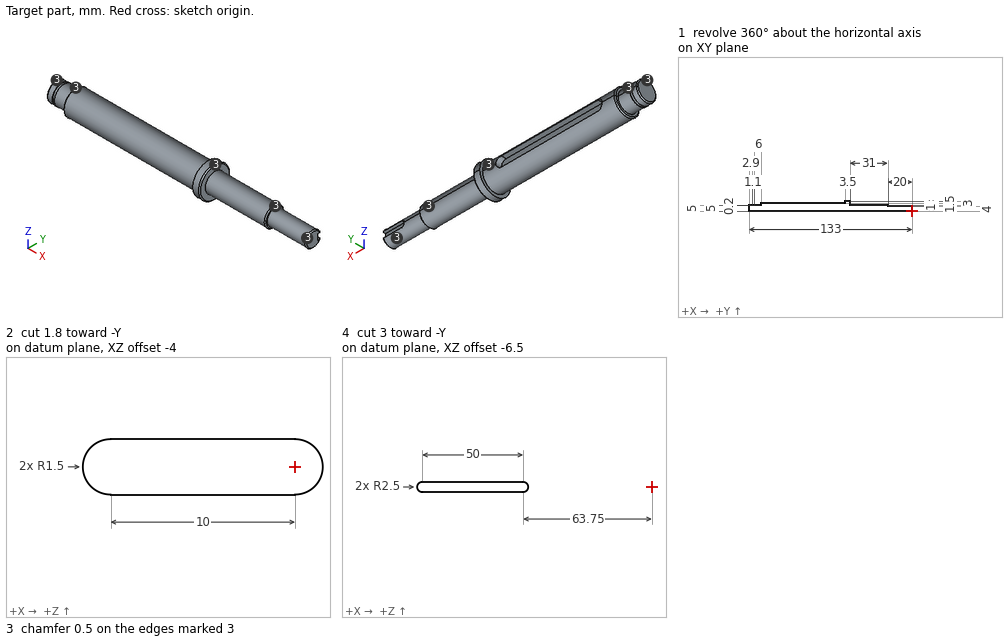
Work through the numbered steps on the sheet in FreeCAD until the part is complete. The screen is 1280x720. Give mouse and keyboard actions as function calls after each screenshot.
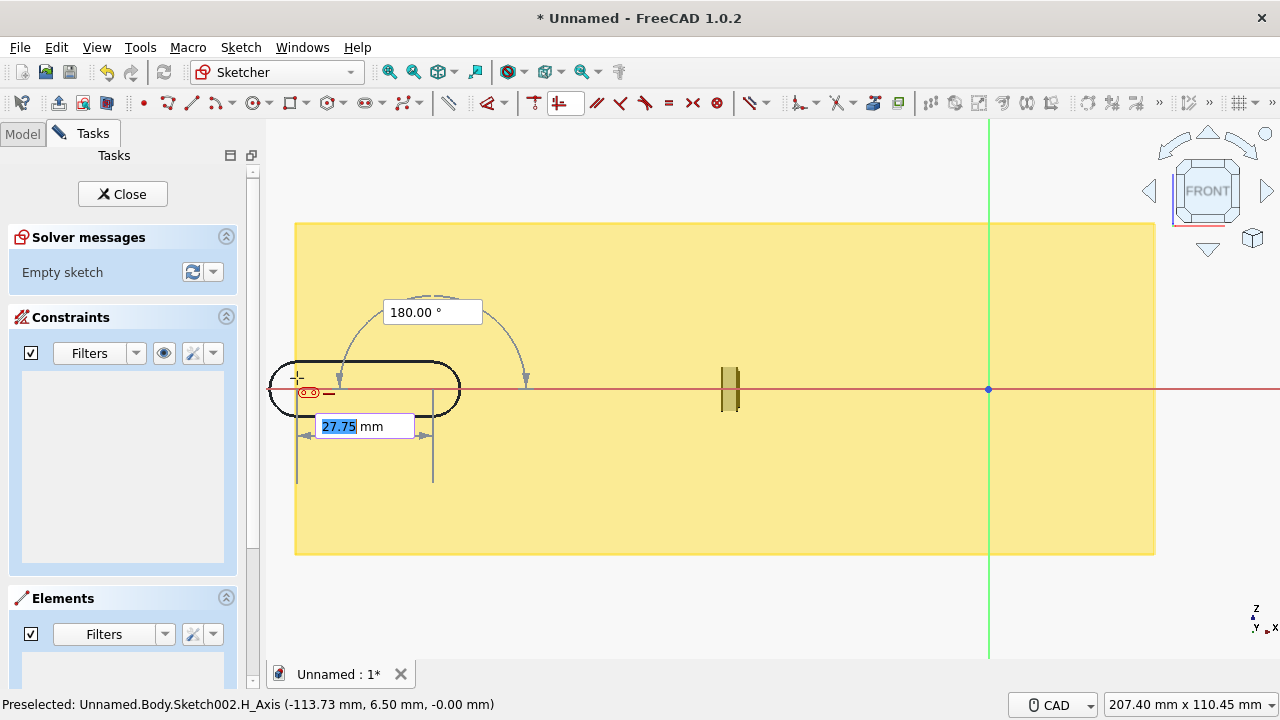
click(677, 380)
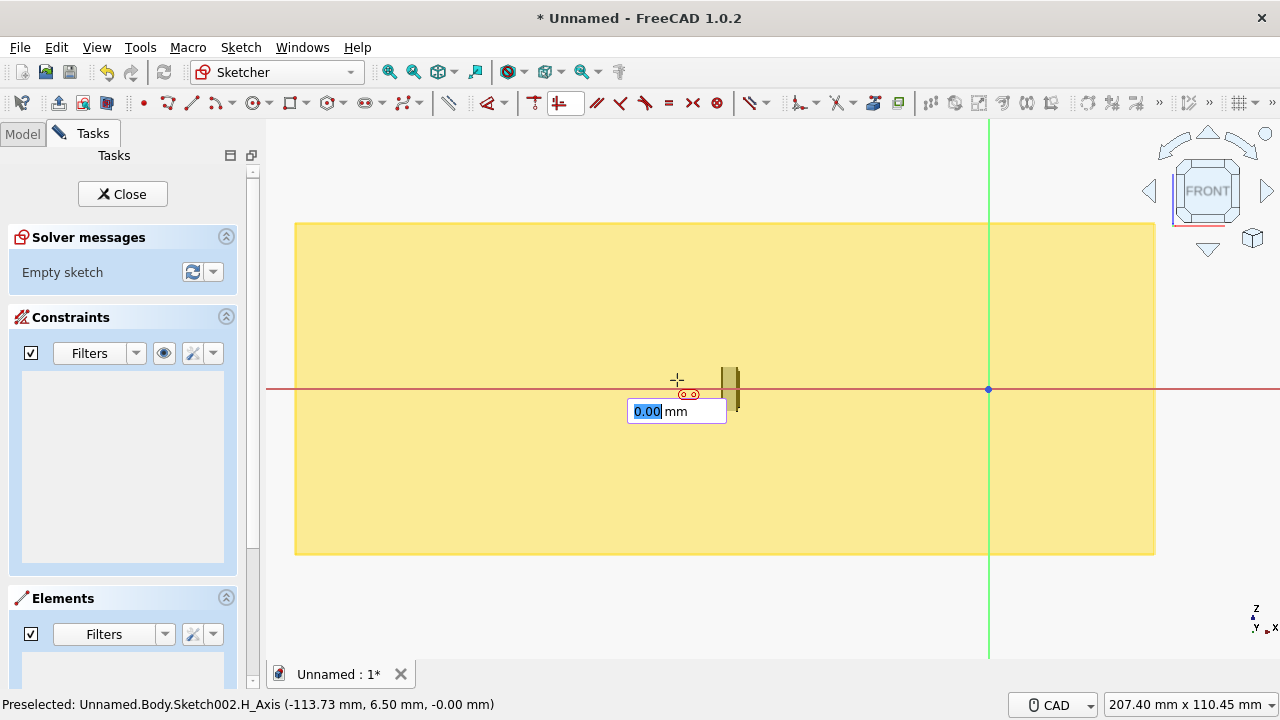
scroll(555, 401, up, 2)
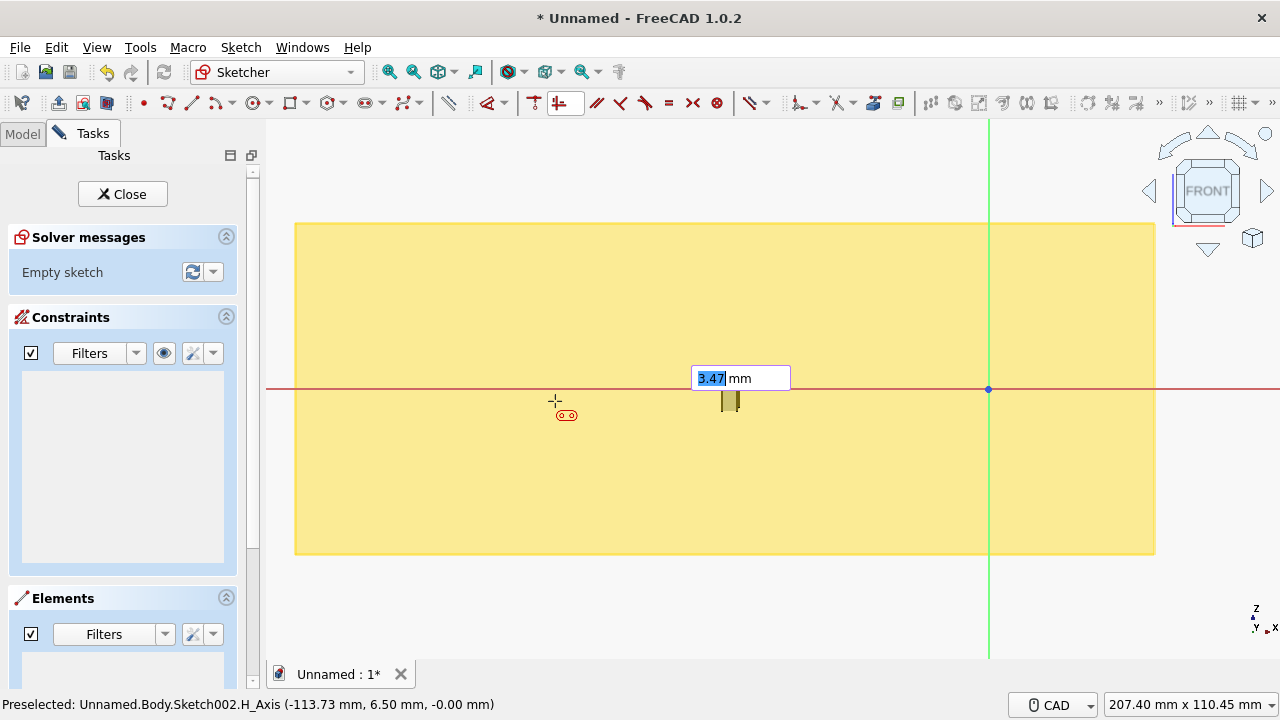
click(555, 401)
key(Escape)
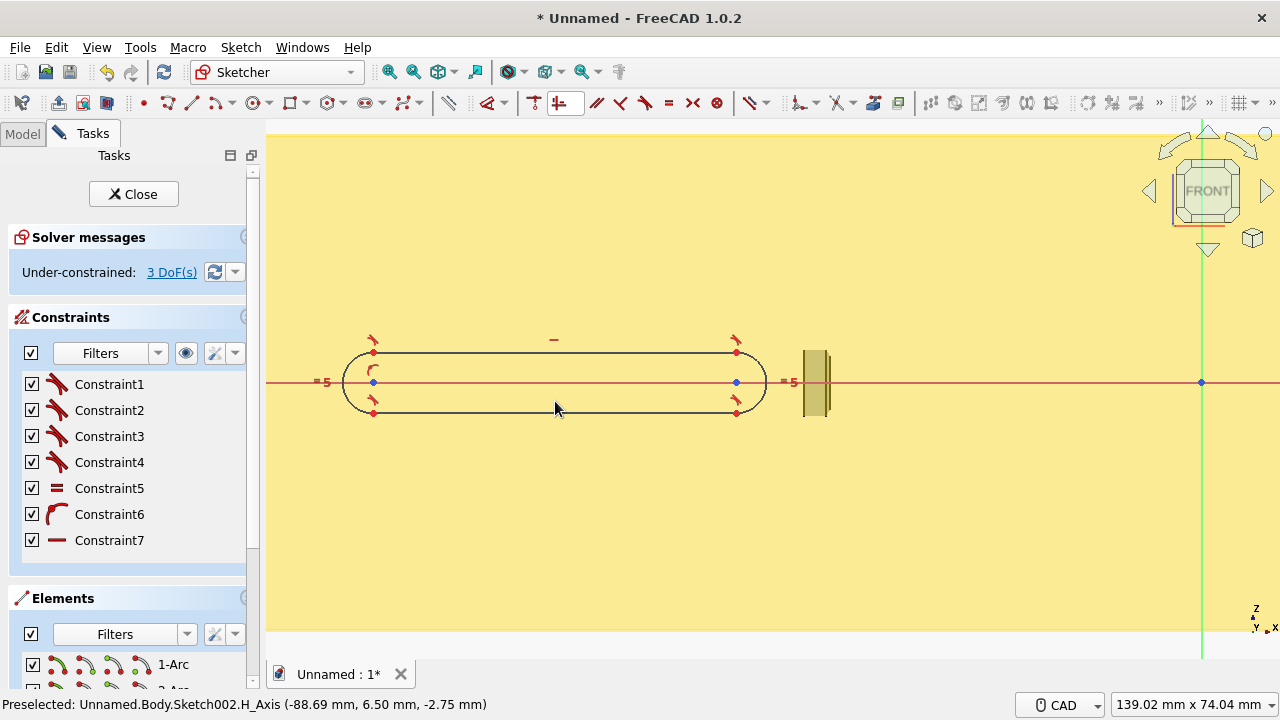
key(d)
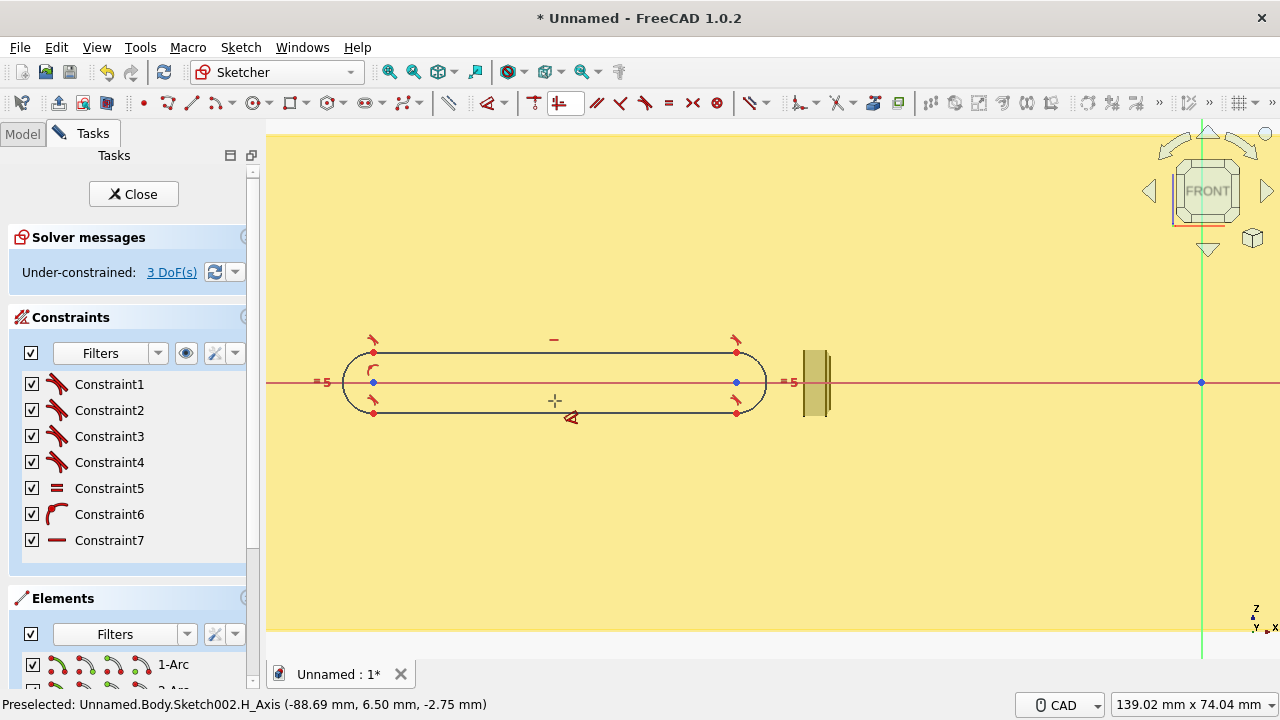
scroll(349, 365, up, 4)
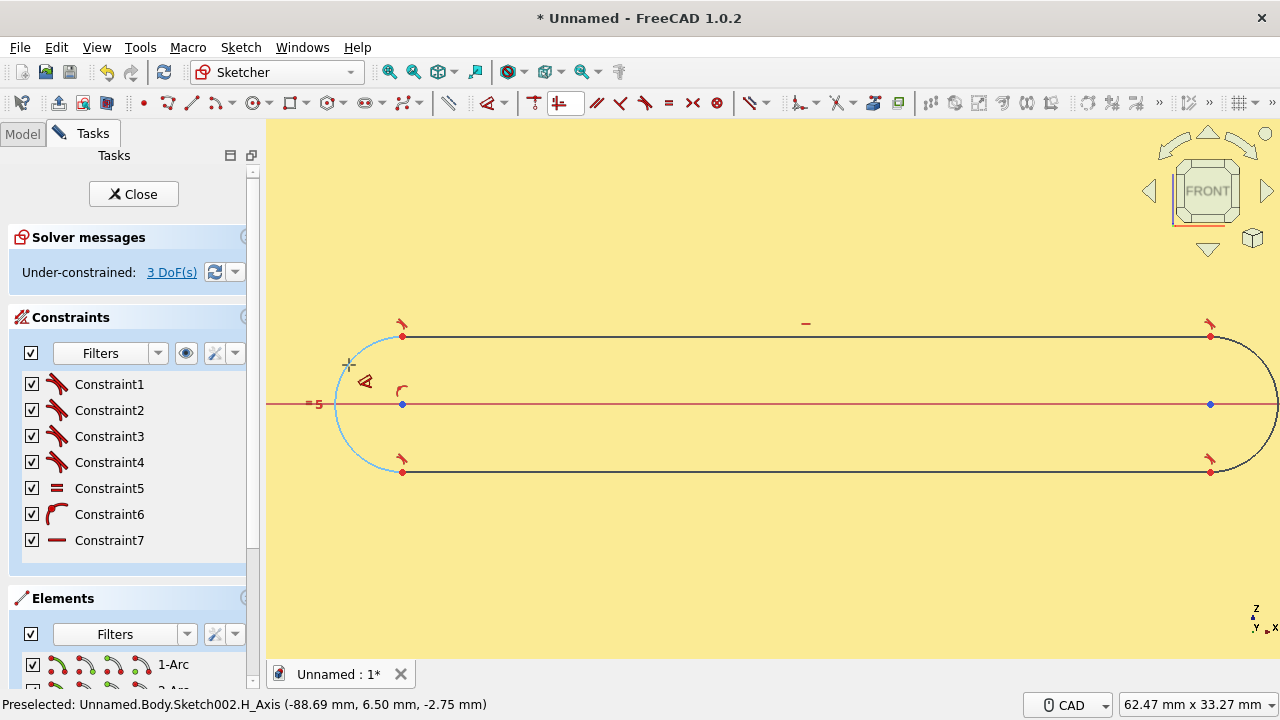
click(348, 365)
click(322, 346)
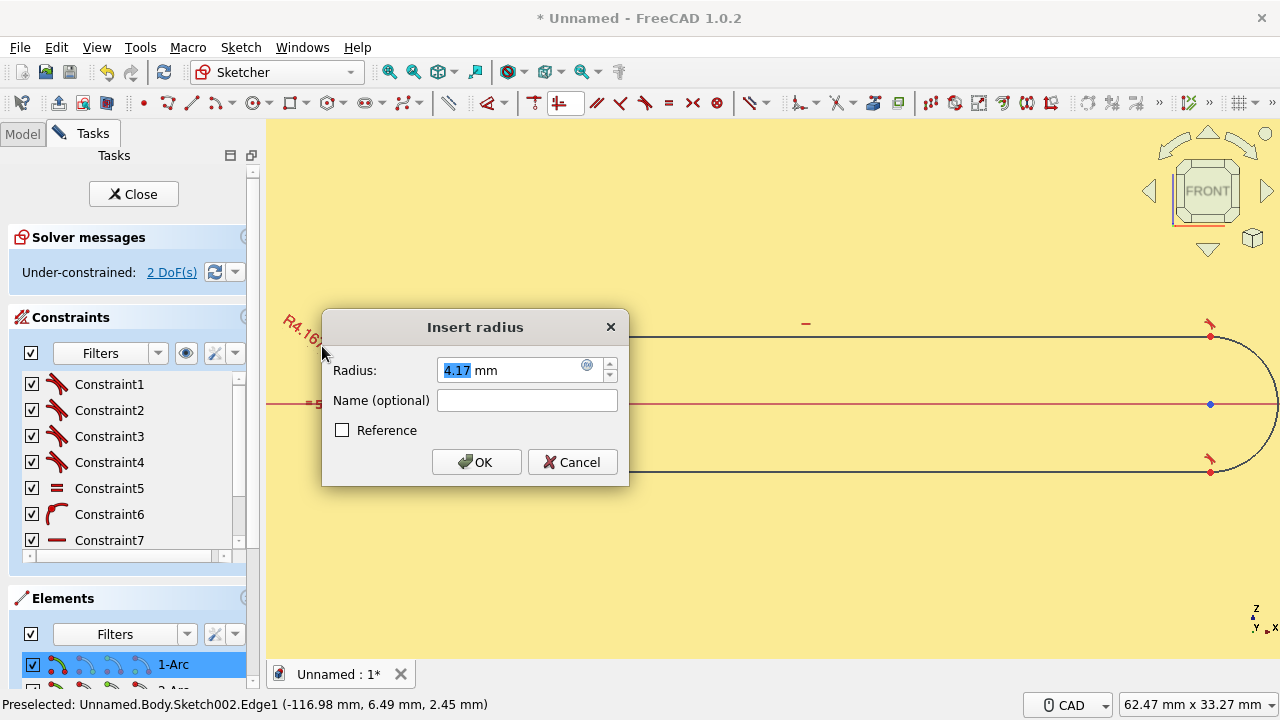
text(2.5)
key(Return)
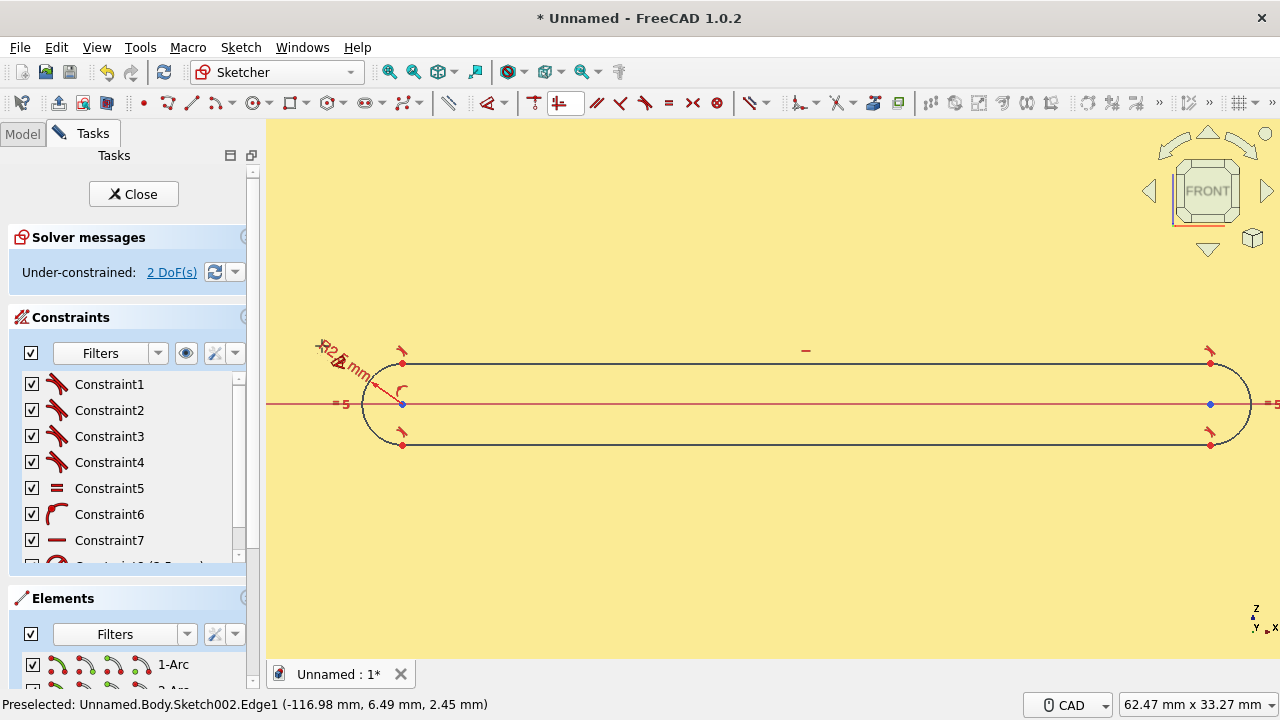
scroll(446, 382, down, 6)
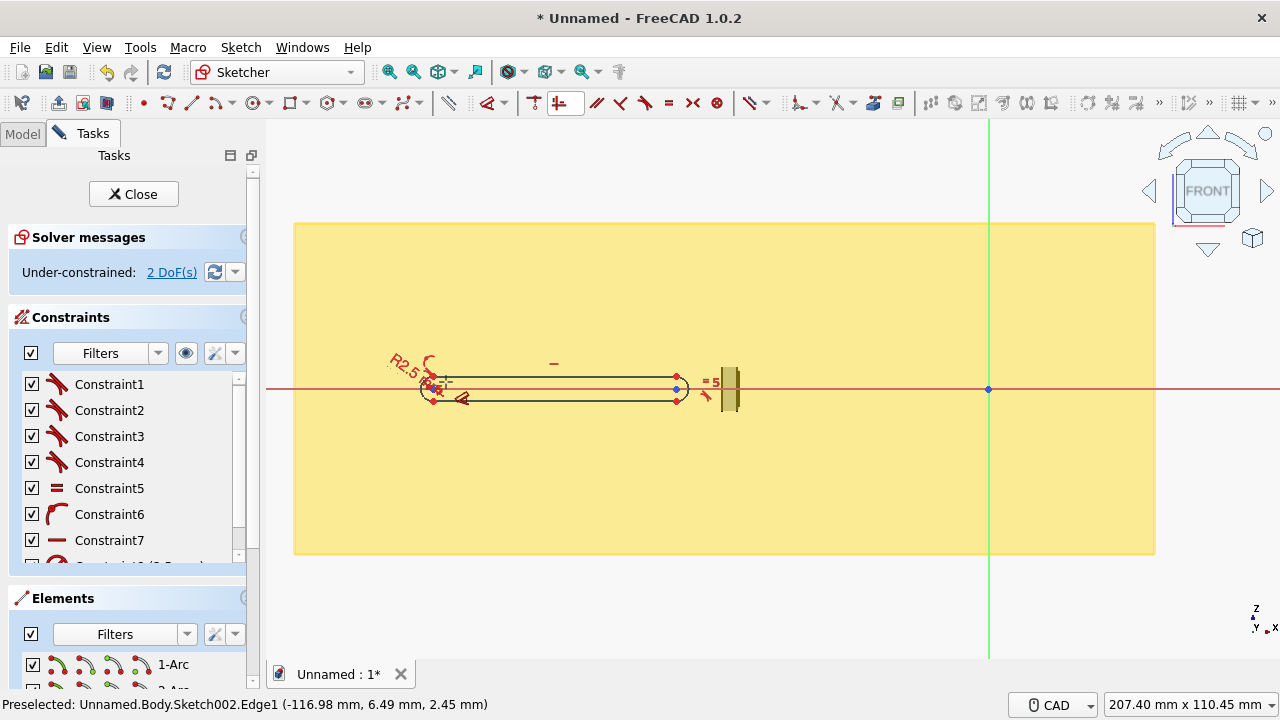
click(506, 377)
click(555, 343)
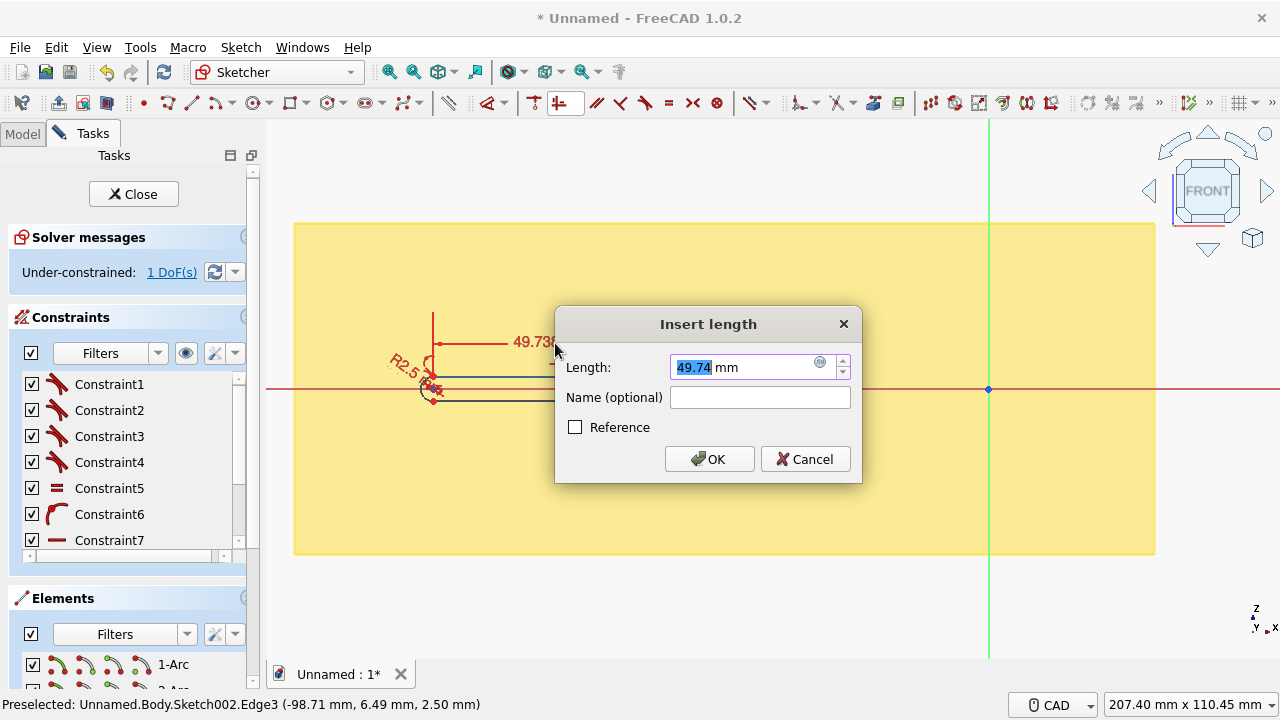
text(50)
key(Return)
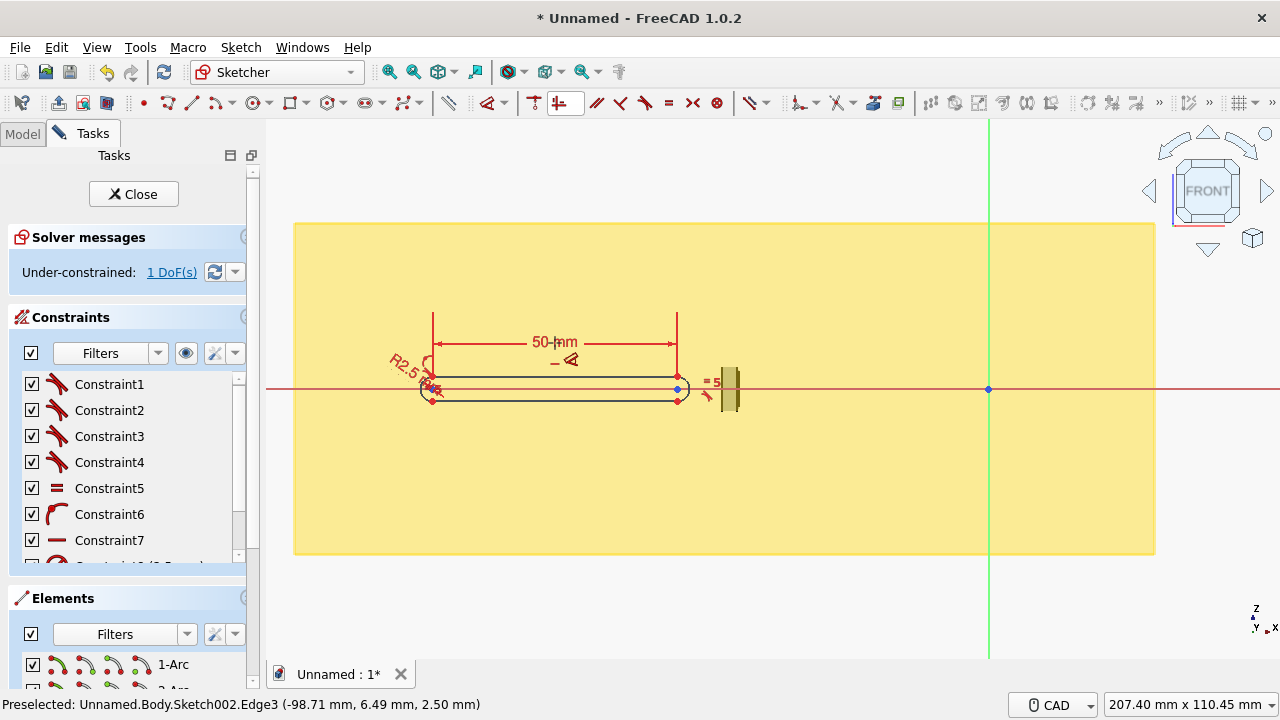
click(677, 401)
click(833, 435)